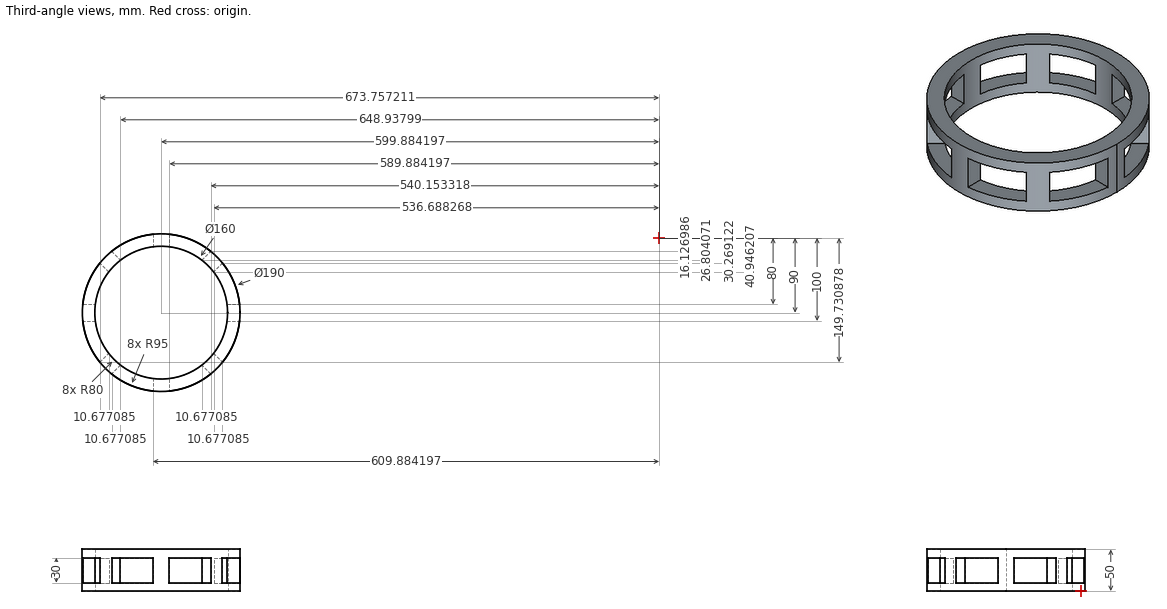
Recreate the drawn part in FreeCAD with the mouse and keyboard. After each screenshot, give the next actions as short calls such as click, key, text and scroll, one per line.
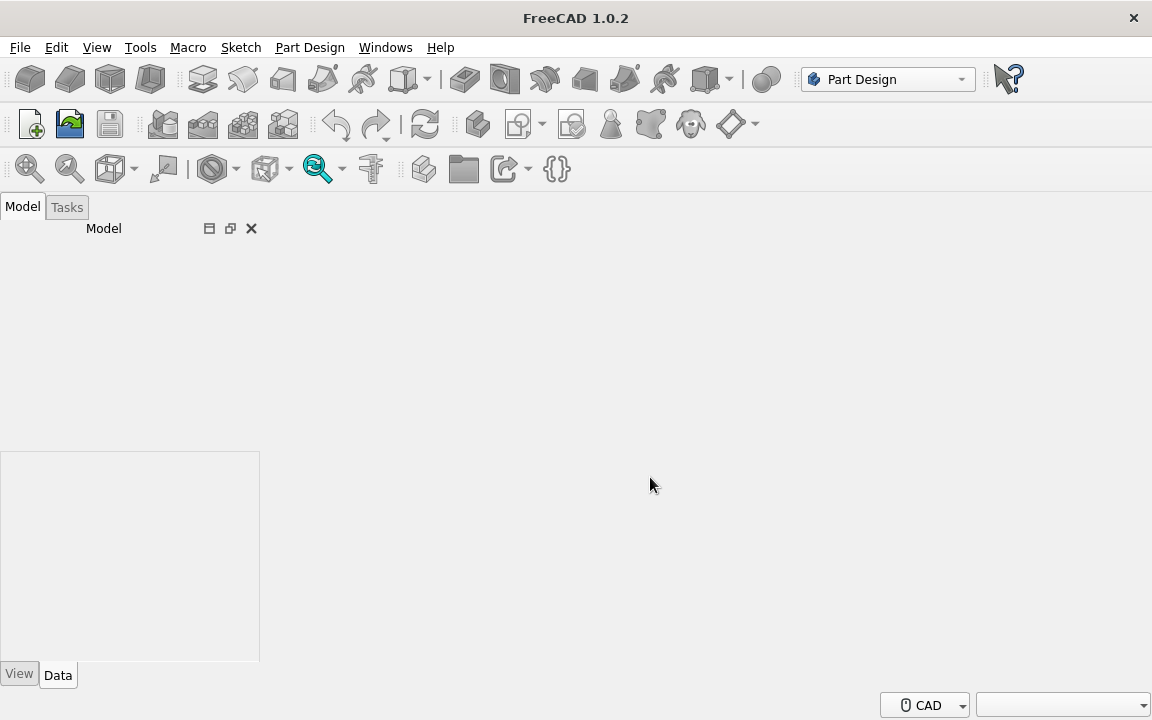
key(ctrl+n)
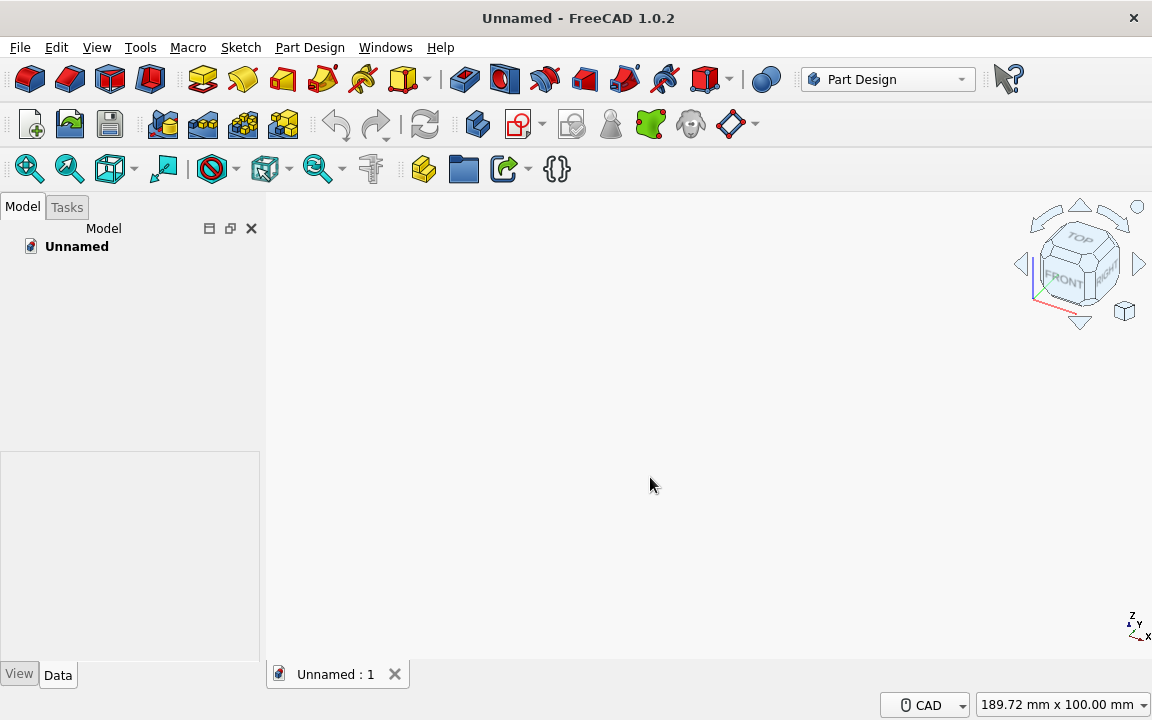
click(518, 124)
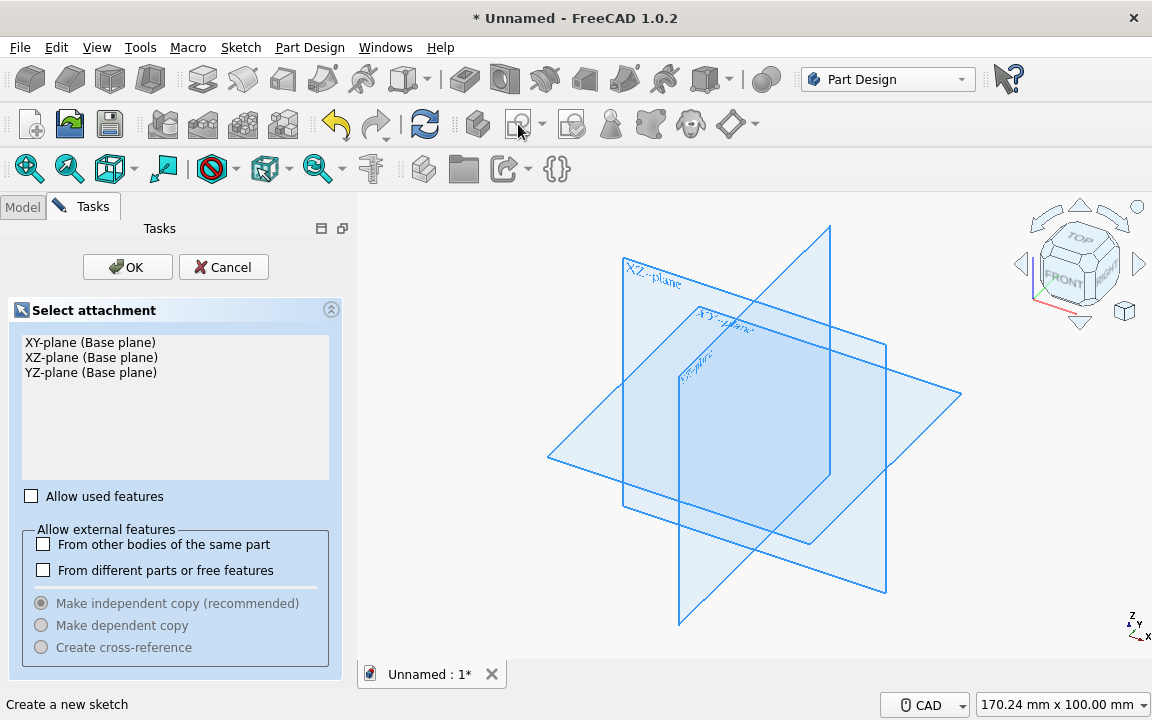
click(82, 342)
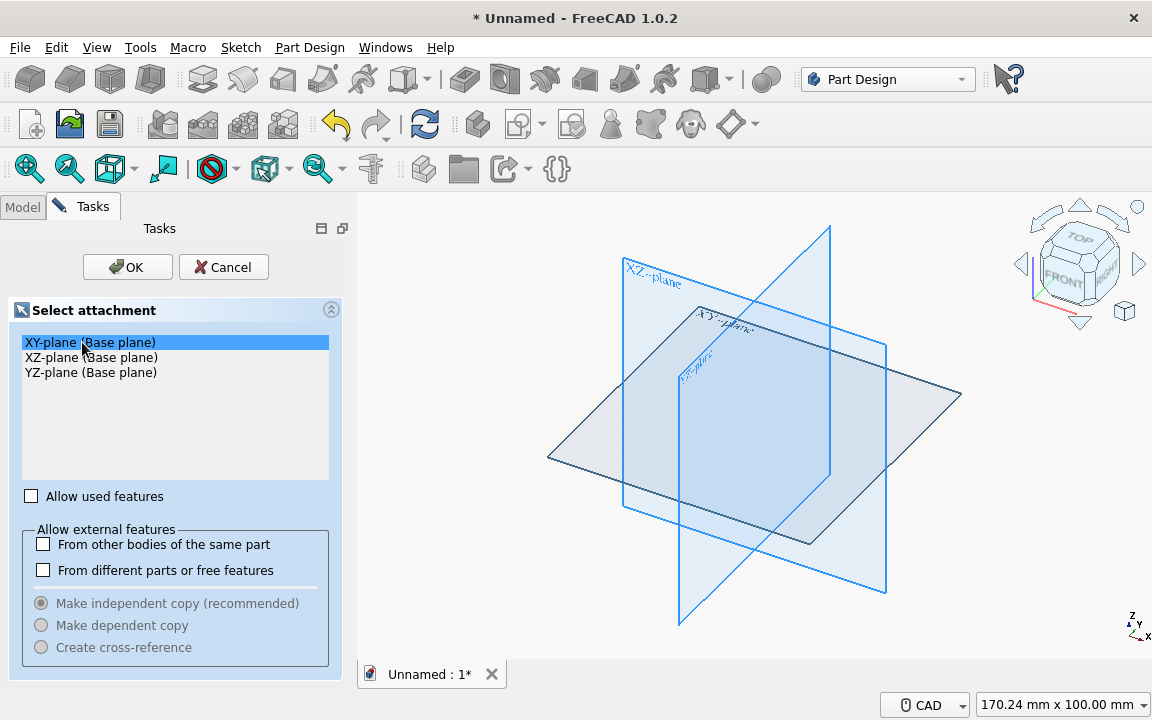
click(128, 267)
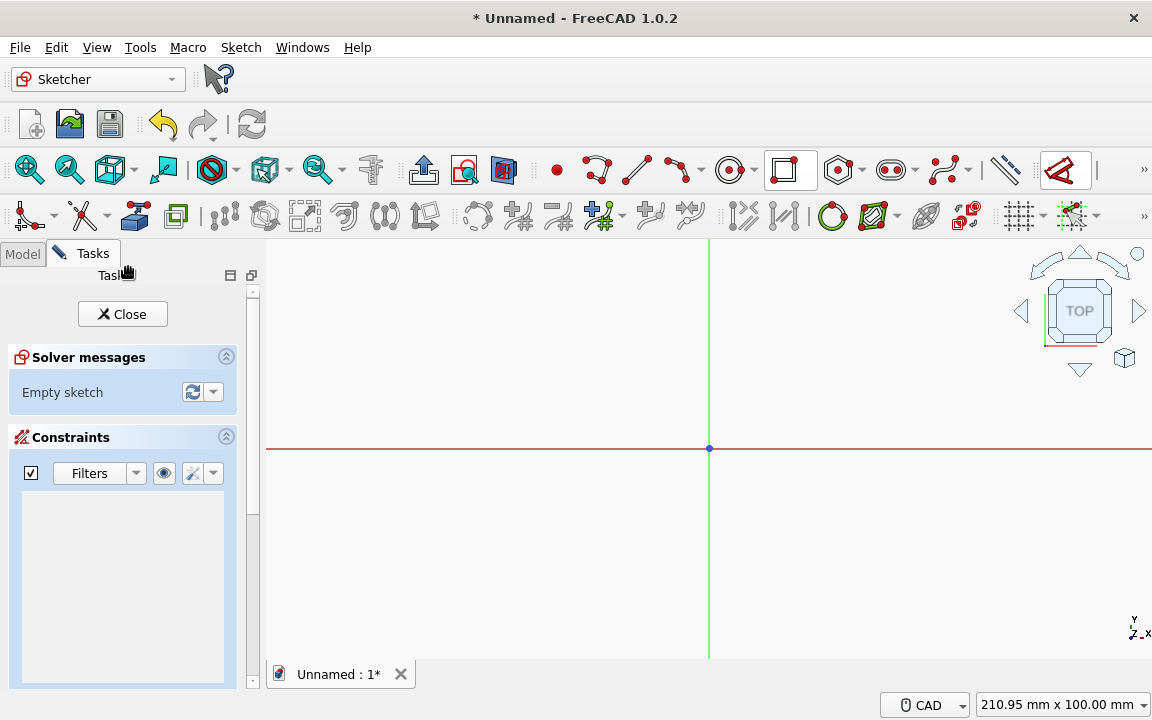
scroll(987, 353, down, 8)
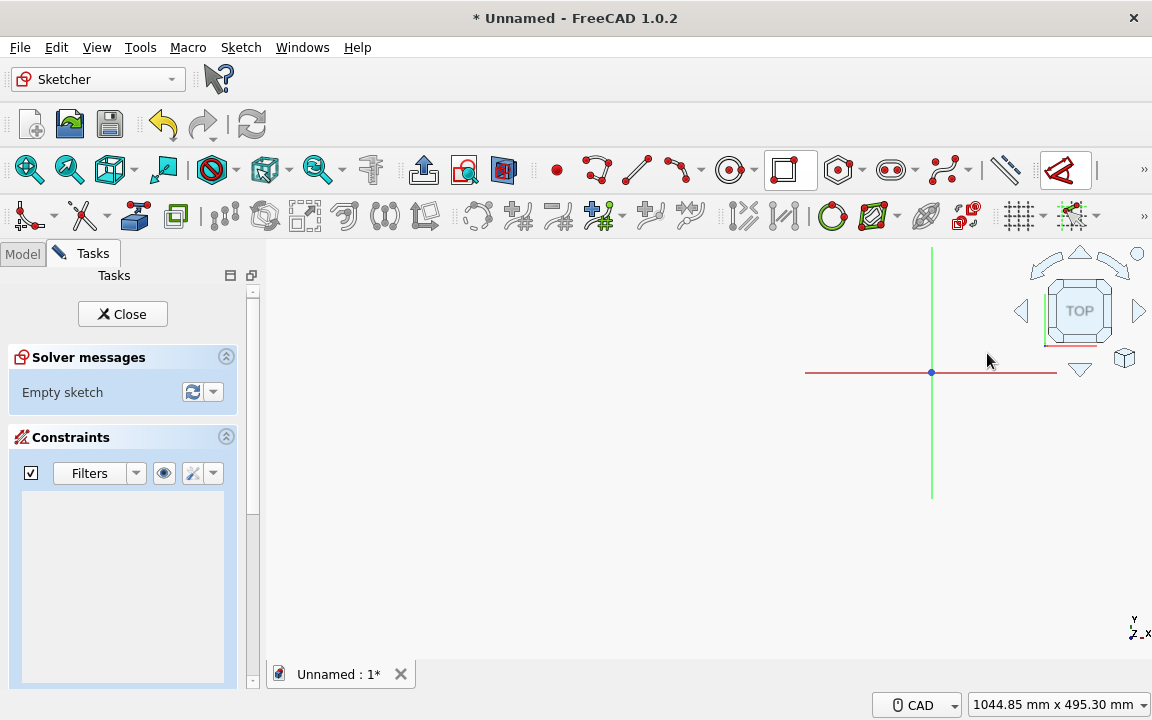
scroll(294, 449, up, 2)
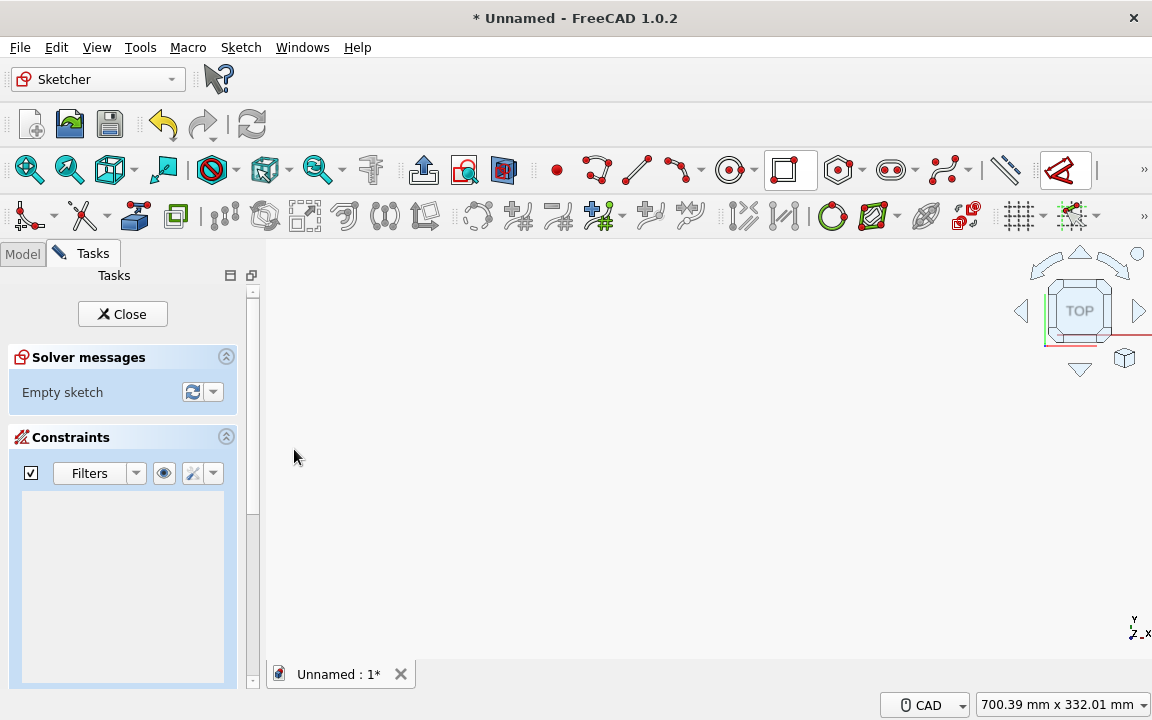
key(g)
key(c)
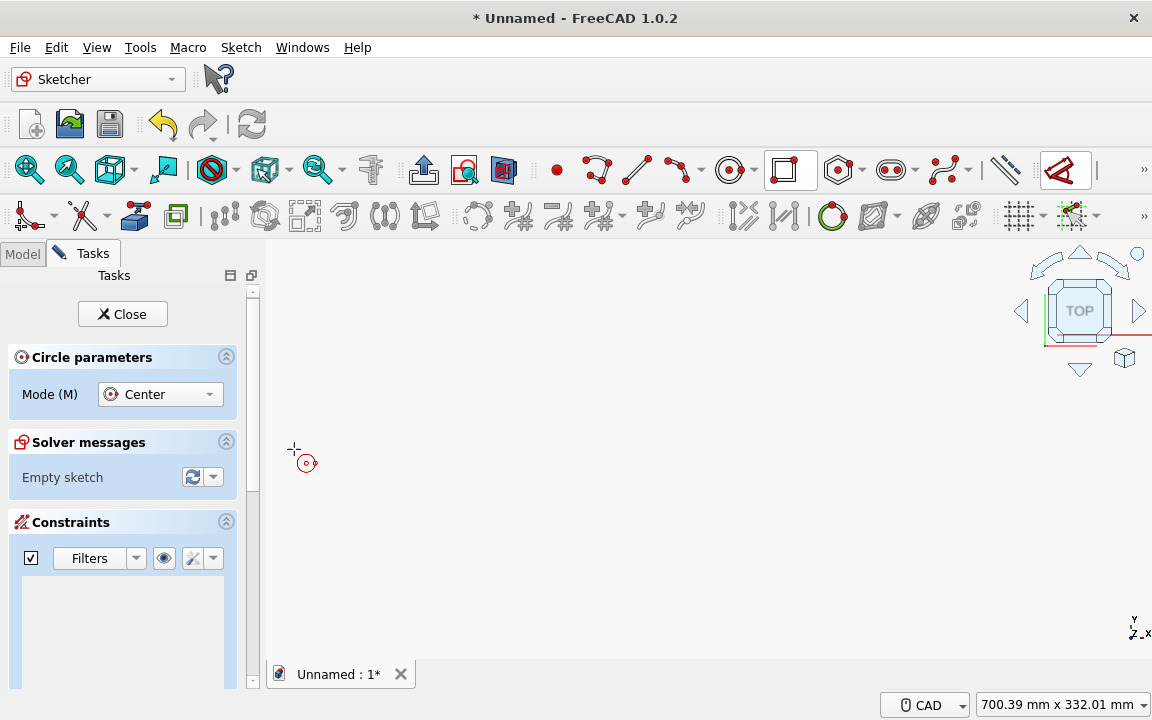
click(486, 449)
click(571, 364)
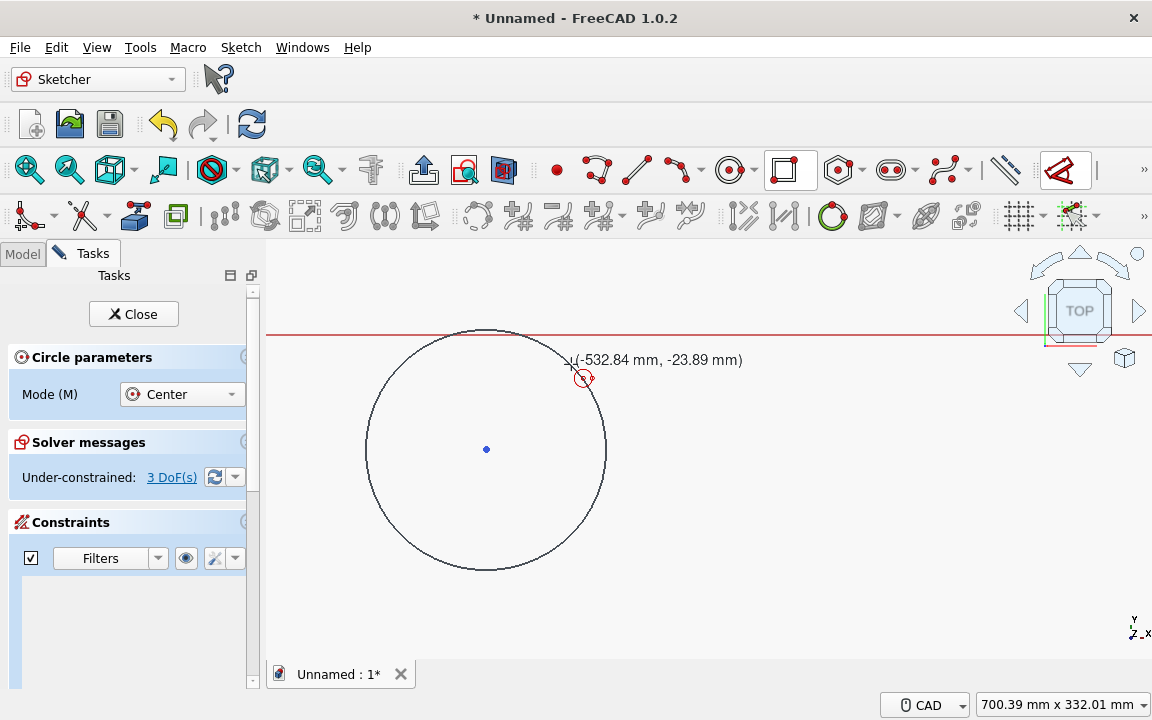
click(486, 450)
click(558, 377)
key(Escape)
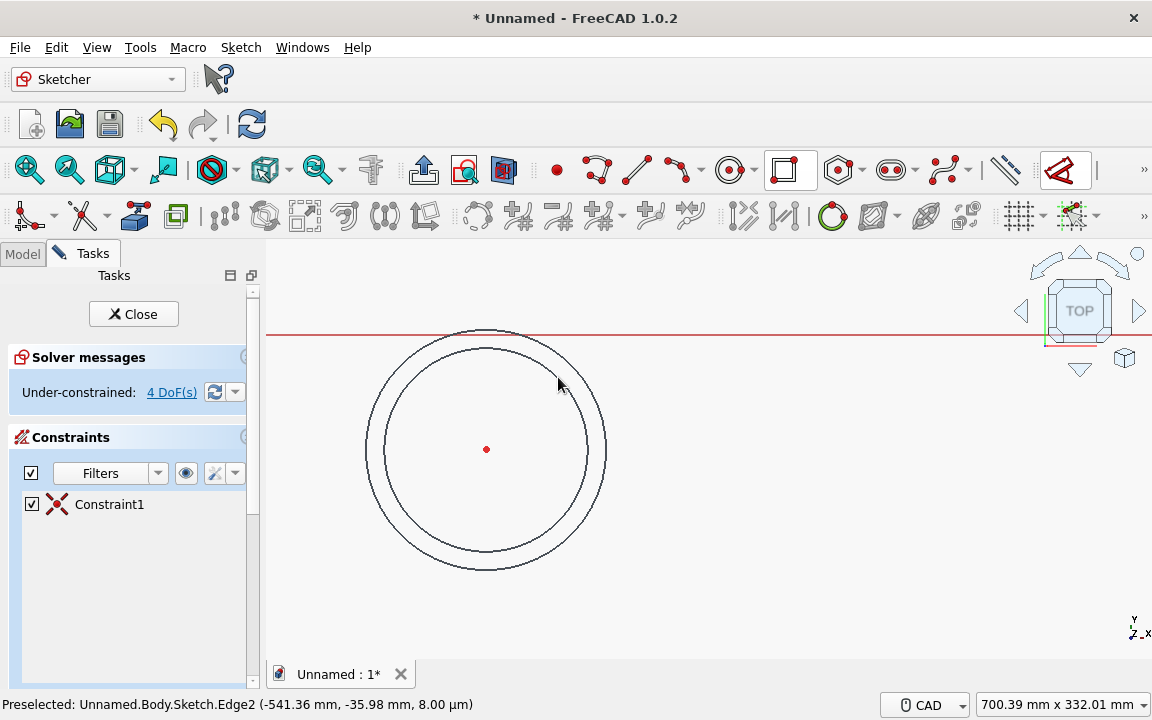
click(571, 365)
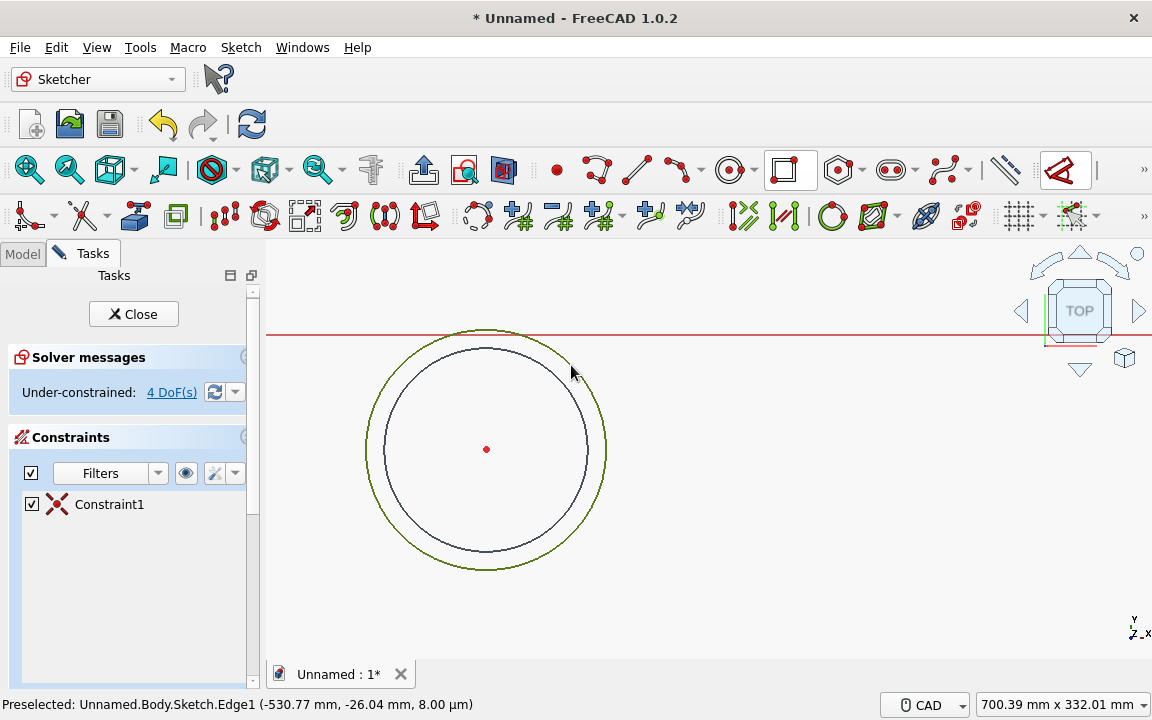
key(k)
key(o)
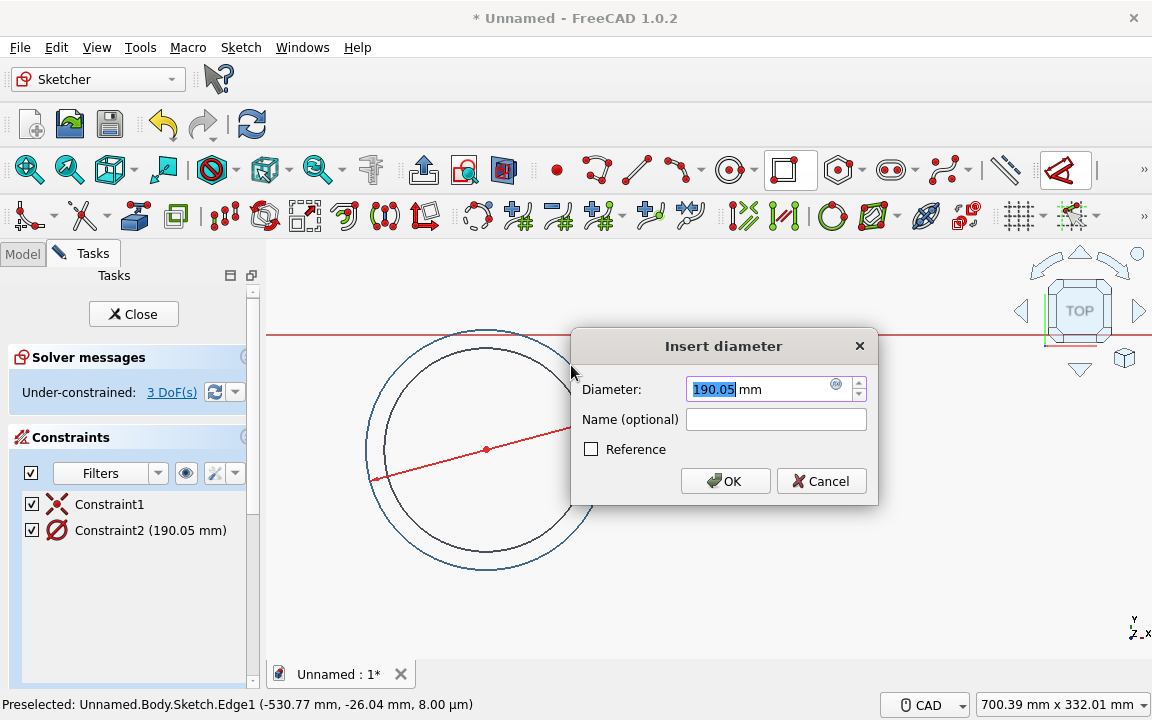
text(190)
key(Return)